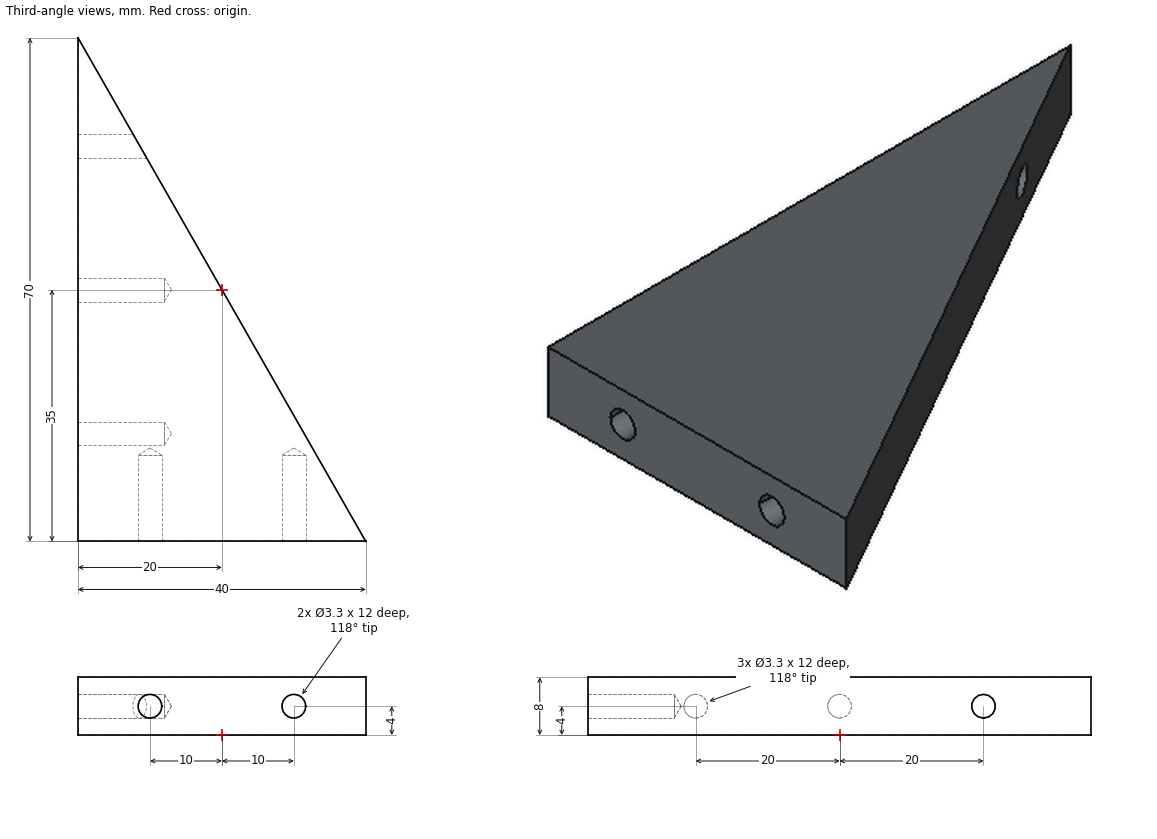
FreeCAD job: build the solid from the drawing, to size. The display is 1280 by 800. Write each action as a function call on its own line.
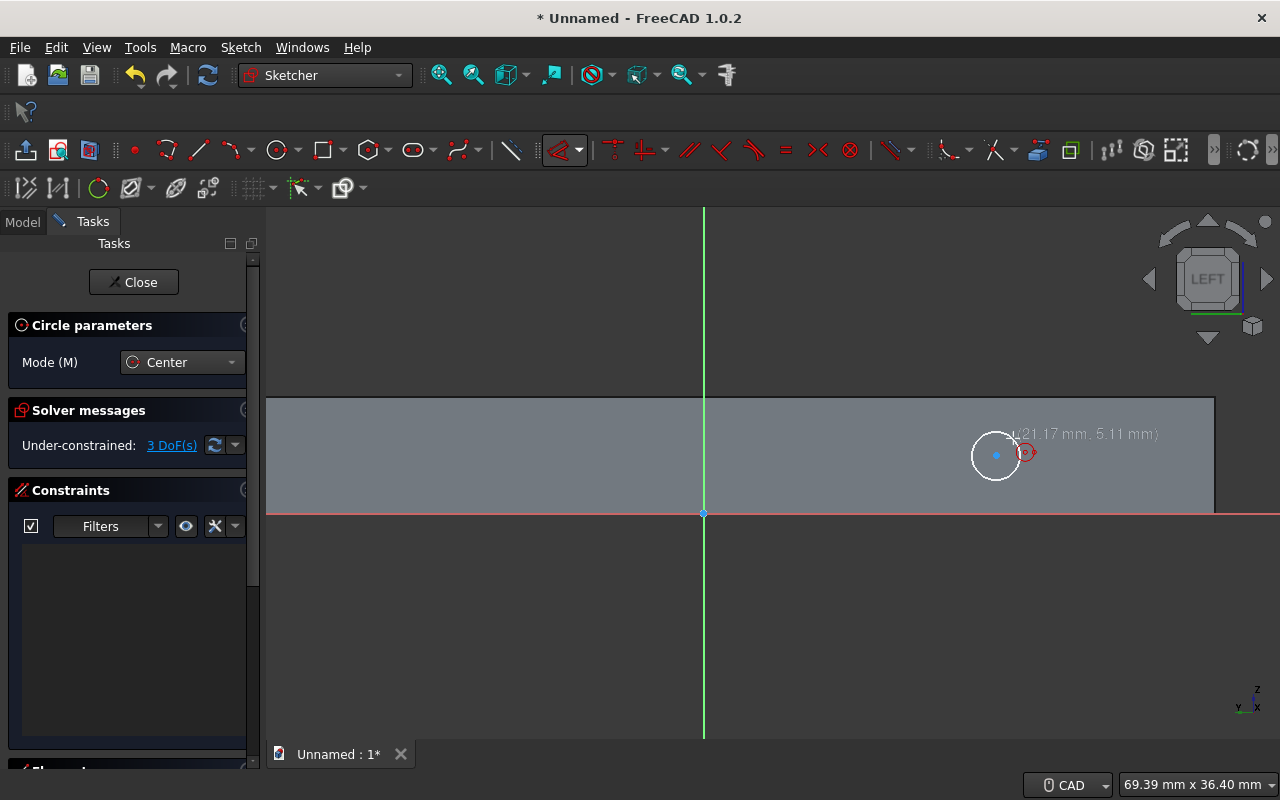
click(704, 455)
click(721, 438)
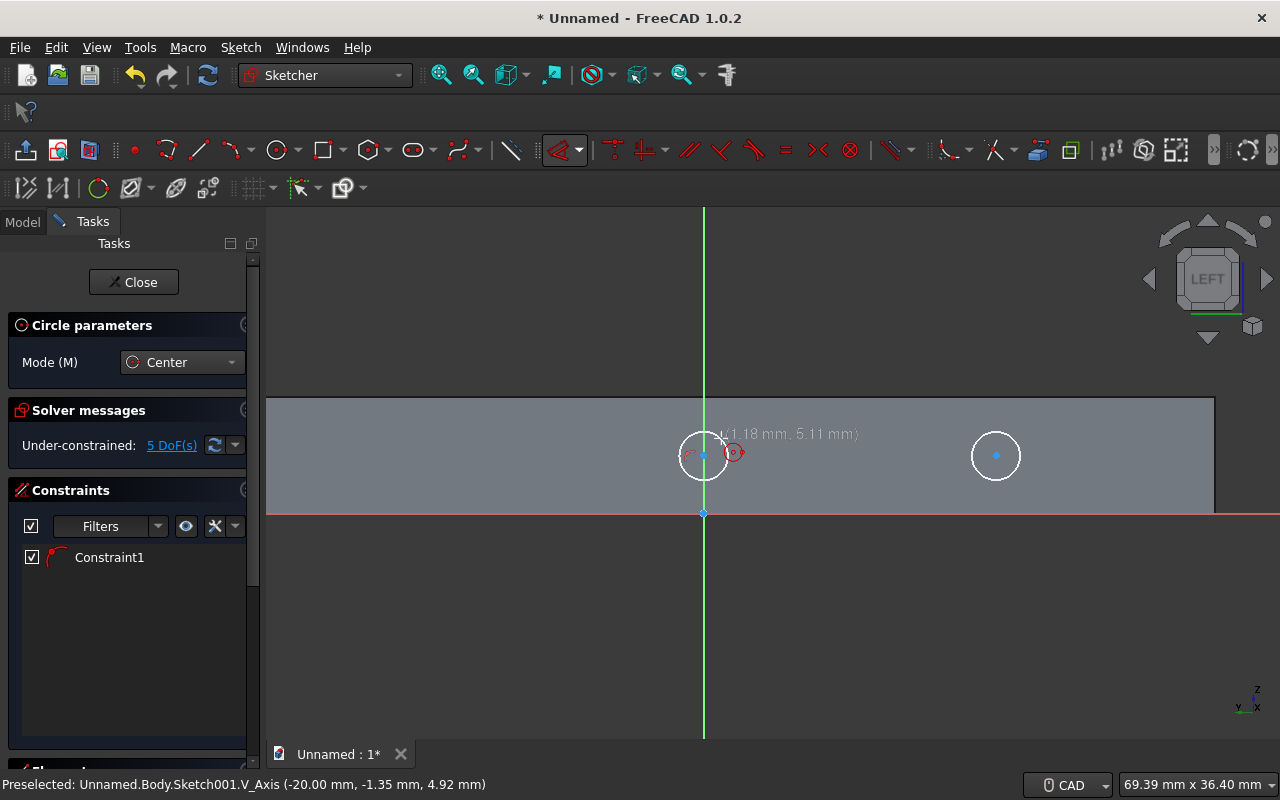
click(411, 455)
click(428, 438)
key(Escape)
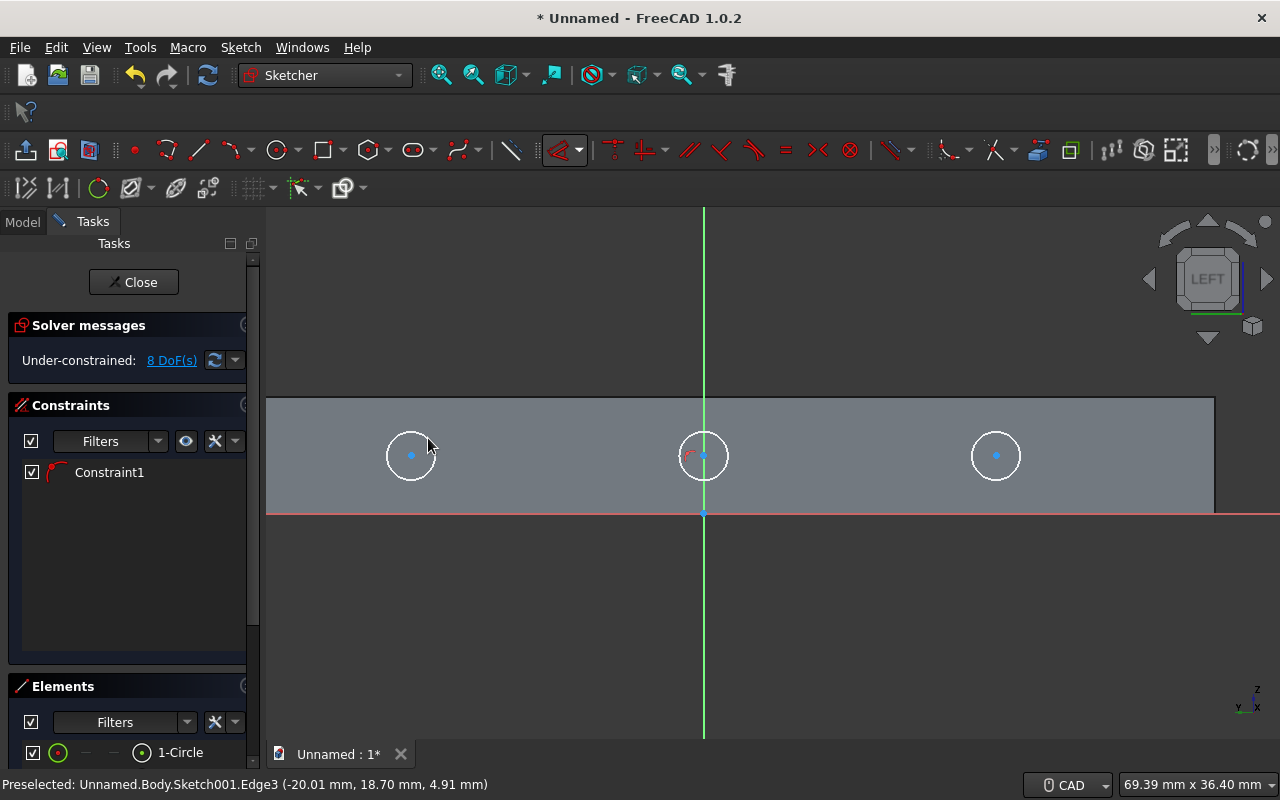
click(1013, 439)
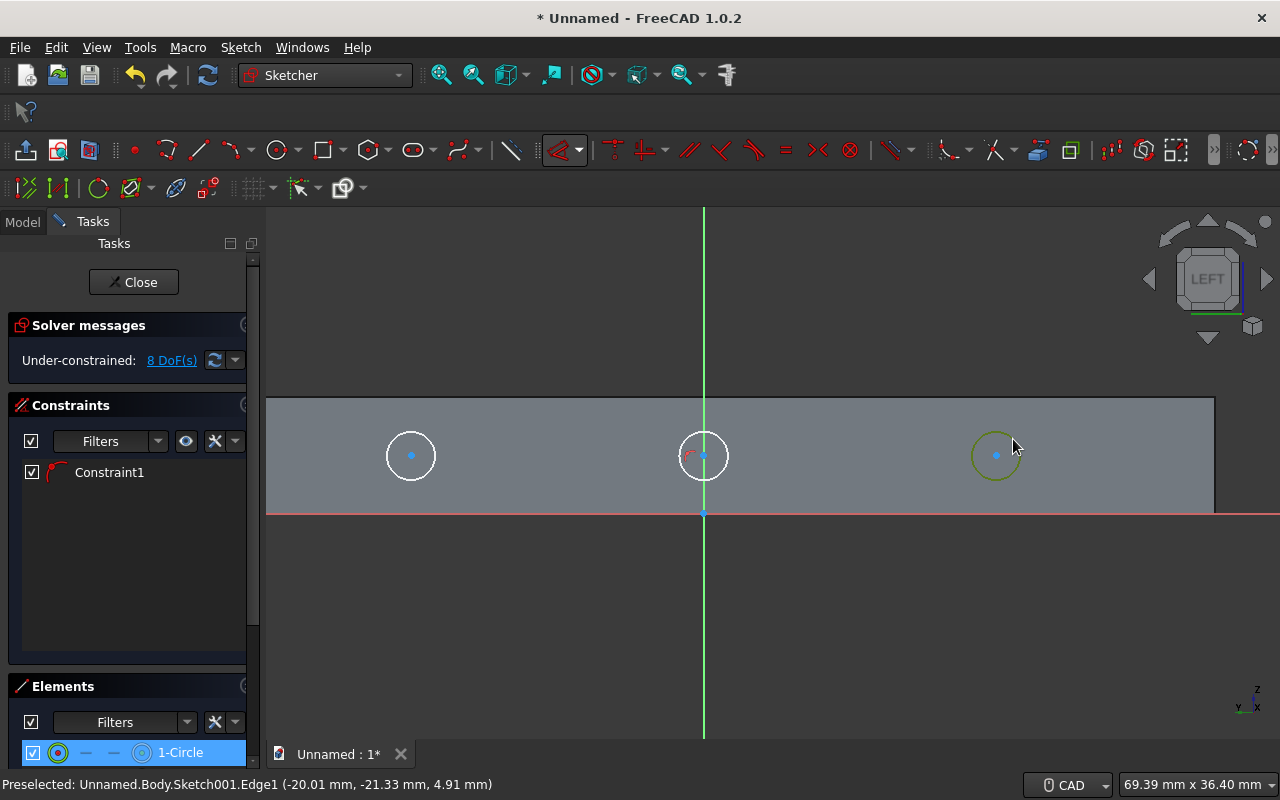
click(721, 439)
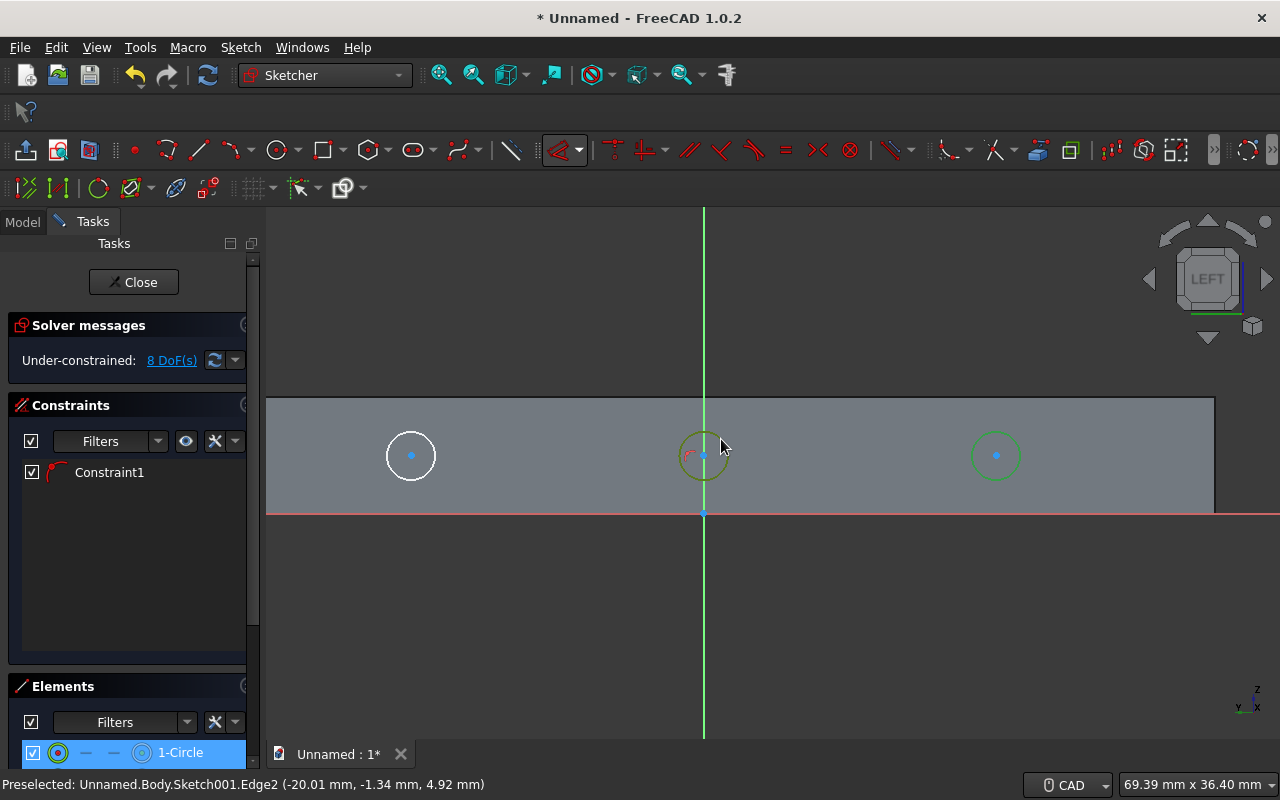
click(428, 439)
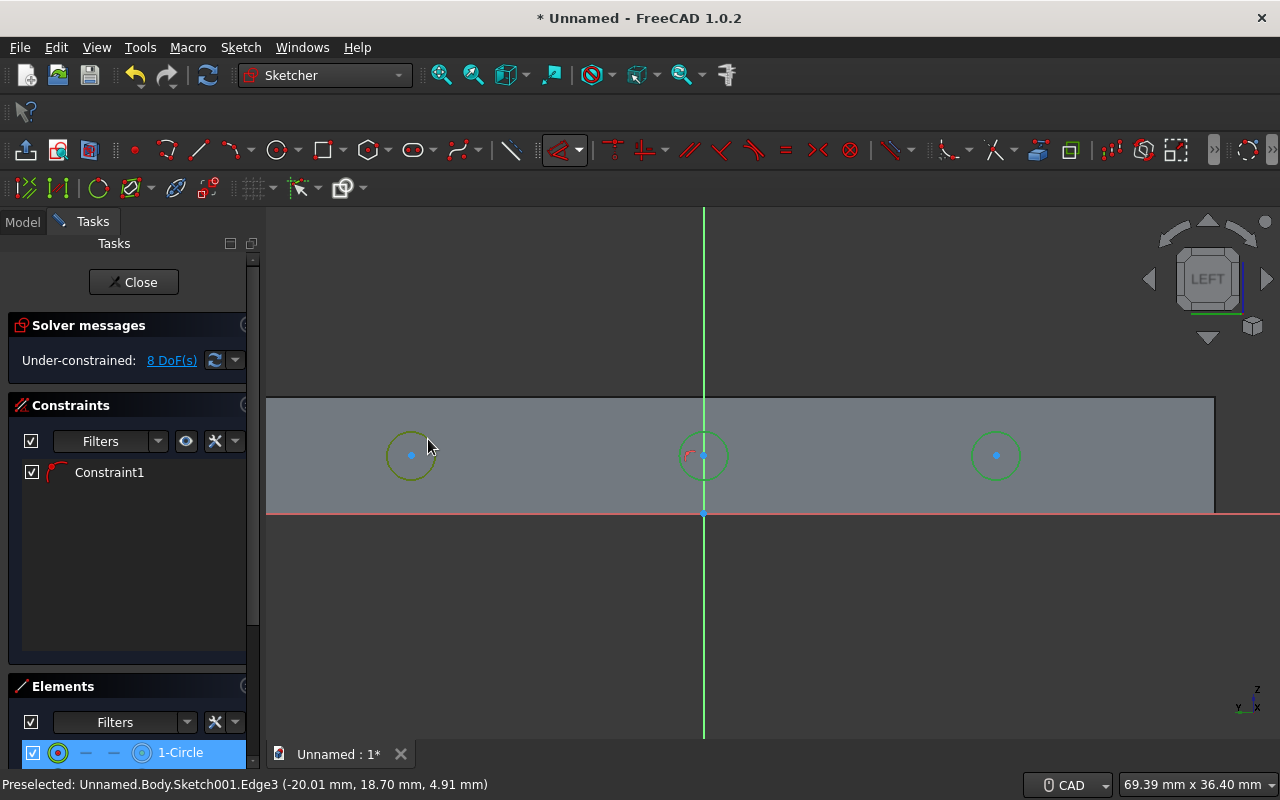
click(786, 150)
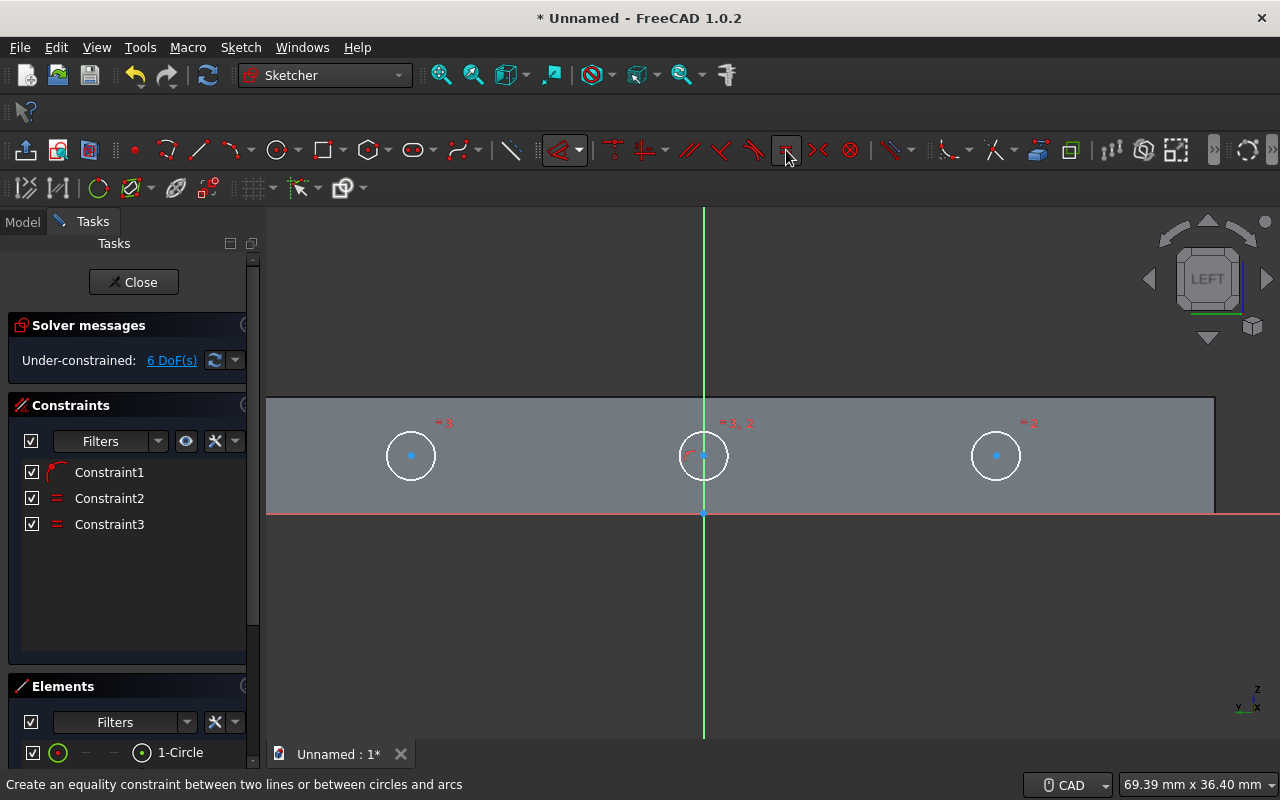
click(996, 456)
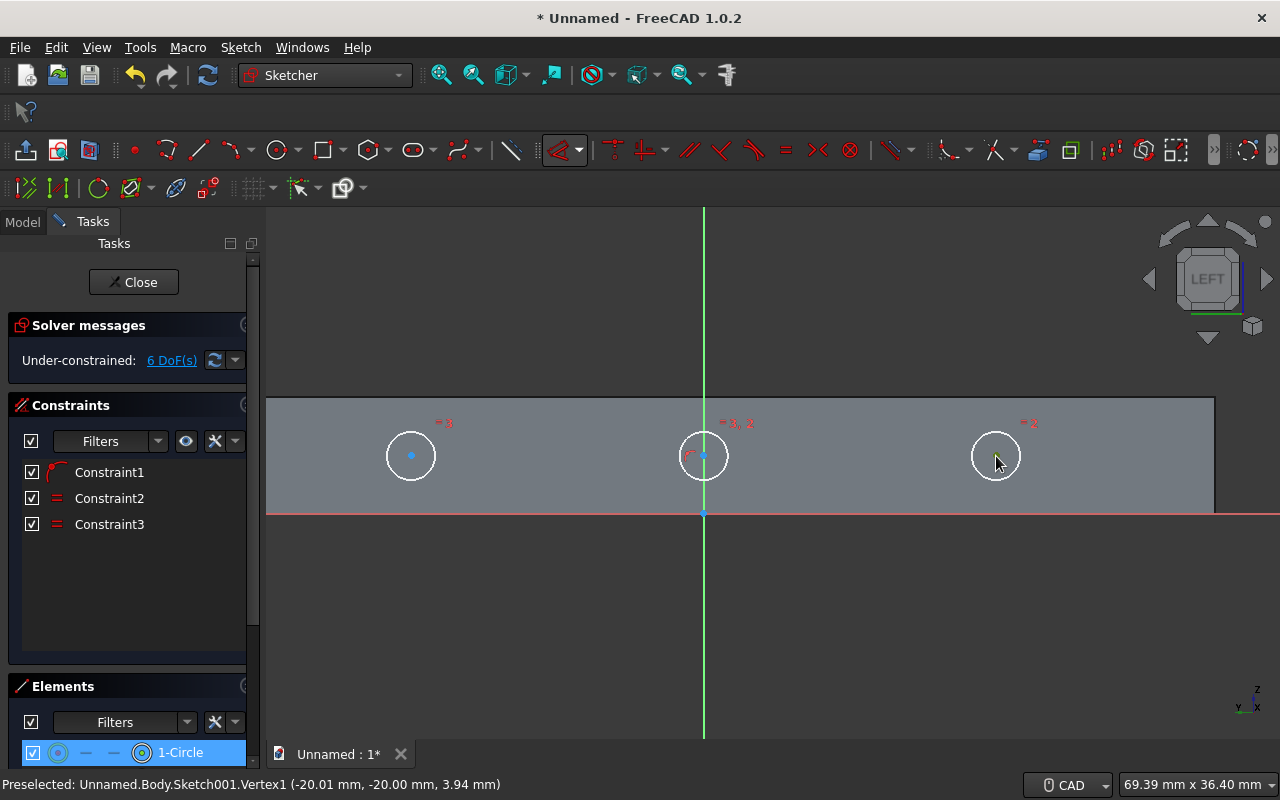
click(704, 456)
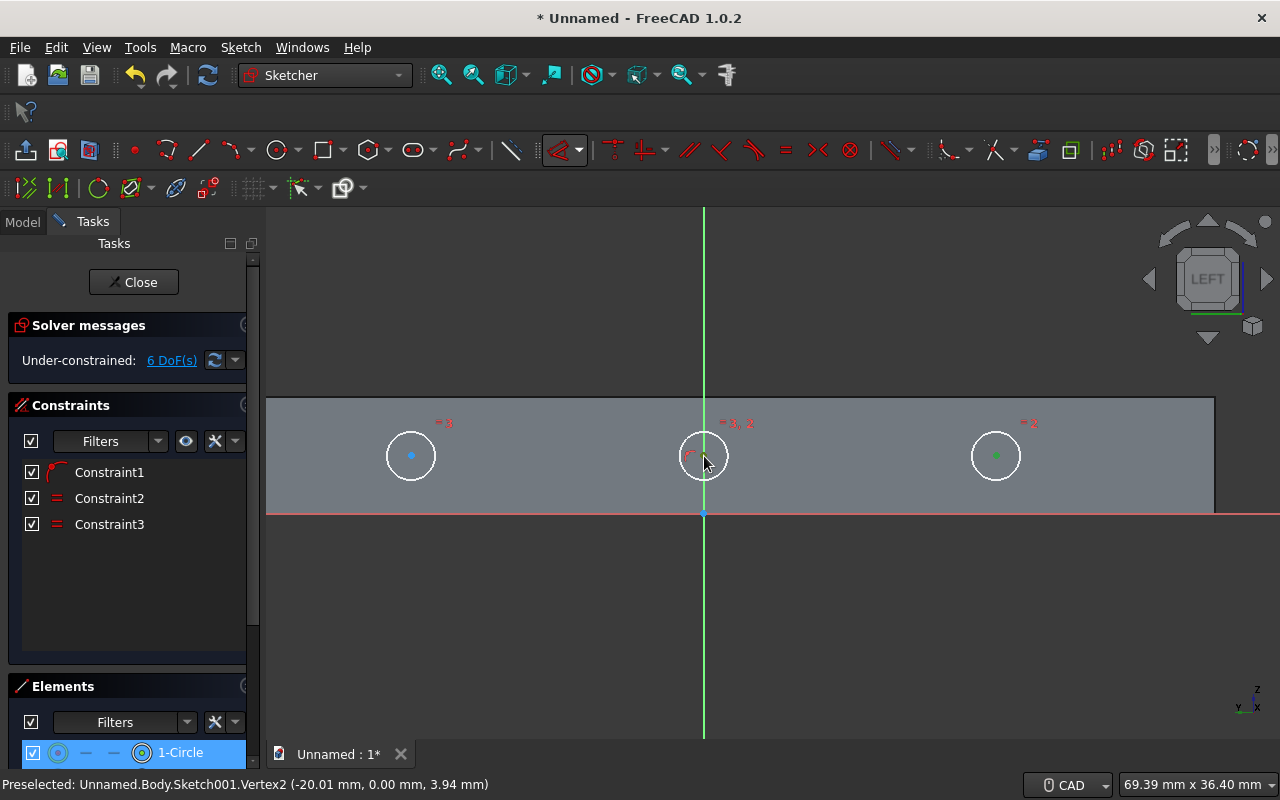
click(668, 150)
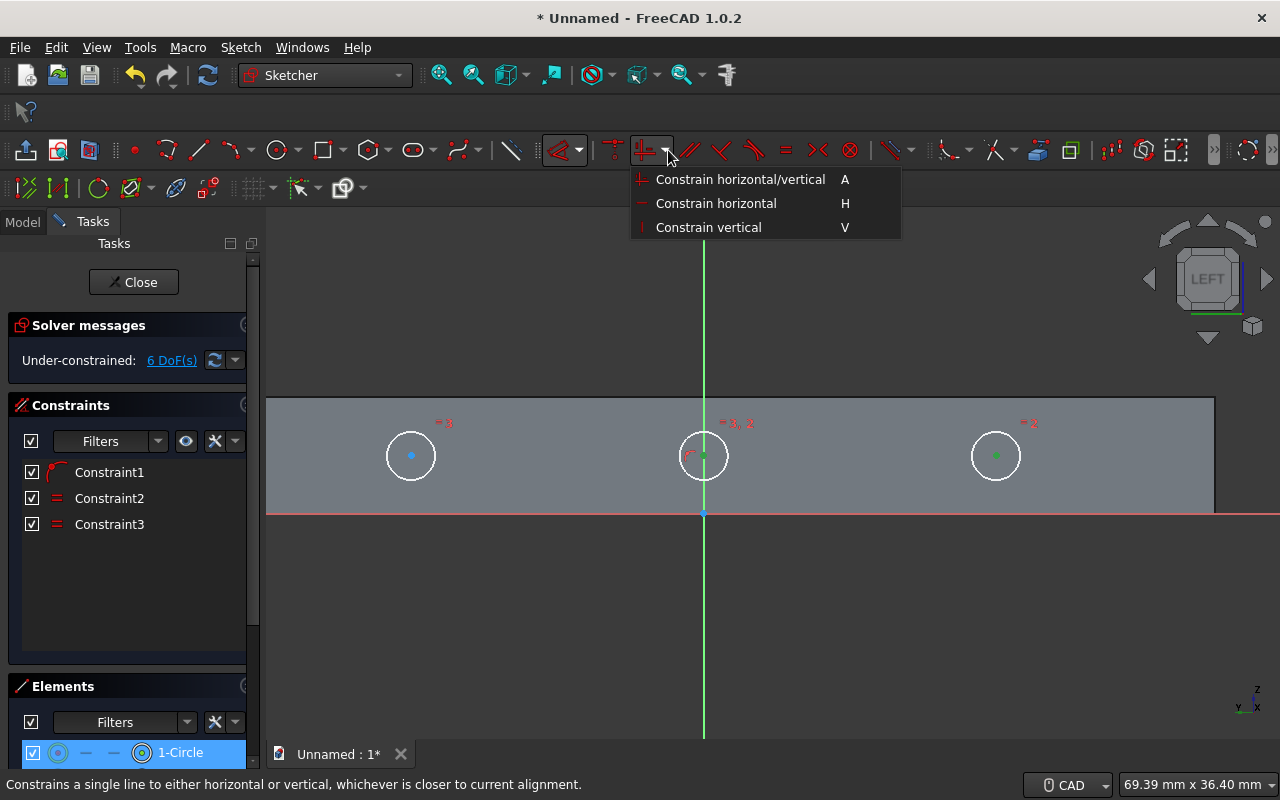
click(766, 203)